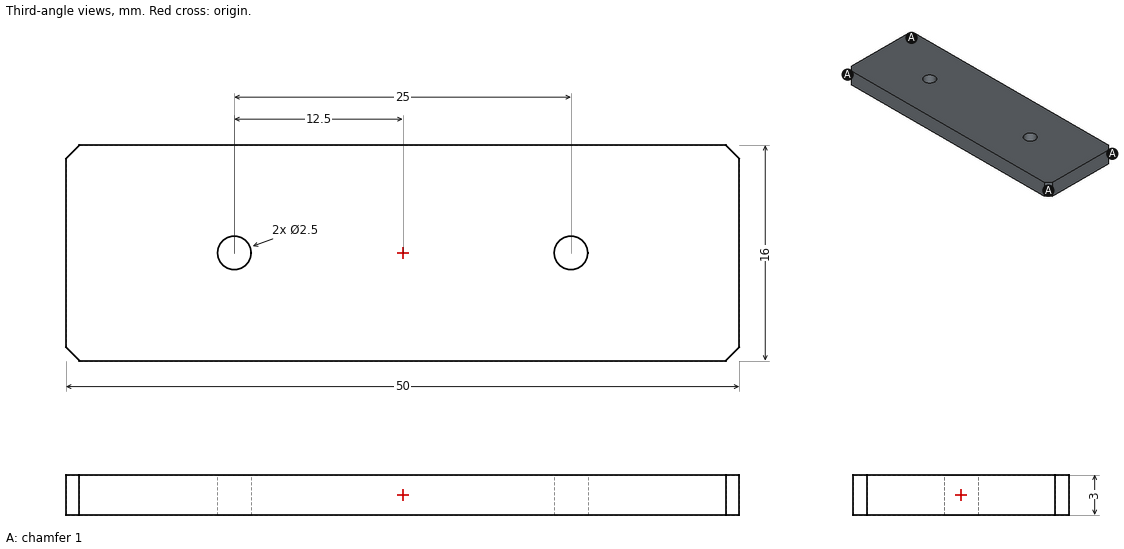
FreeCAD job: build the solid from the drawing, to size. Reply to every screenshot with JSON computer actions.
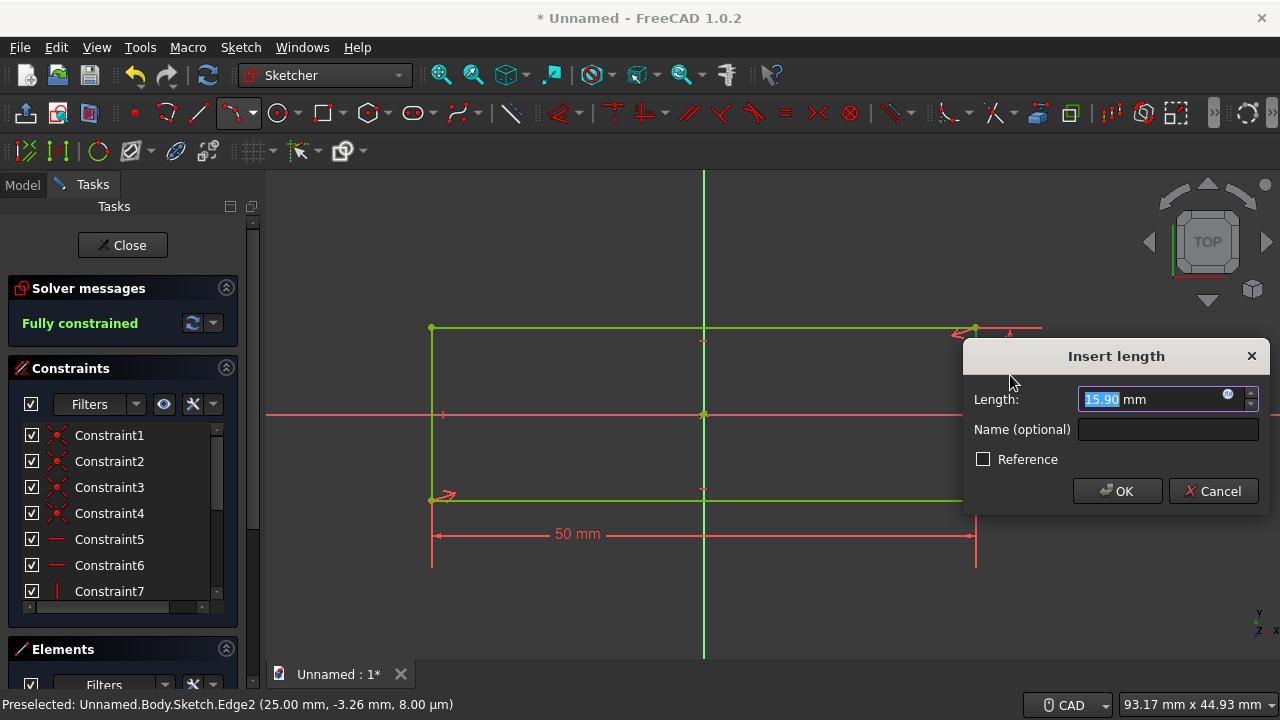
{"action": "type", "text": "16"}
{"action": "key", "text": "Return"}
{"action": "key", "text": "Escape"}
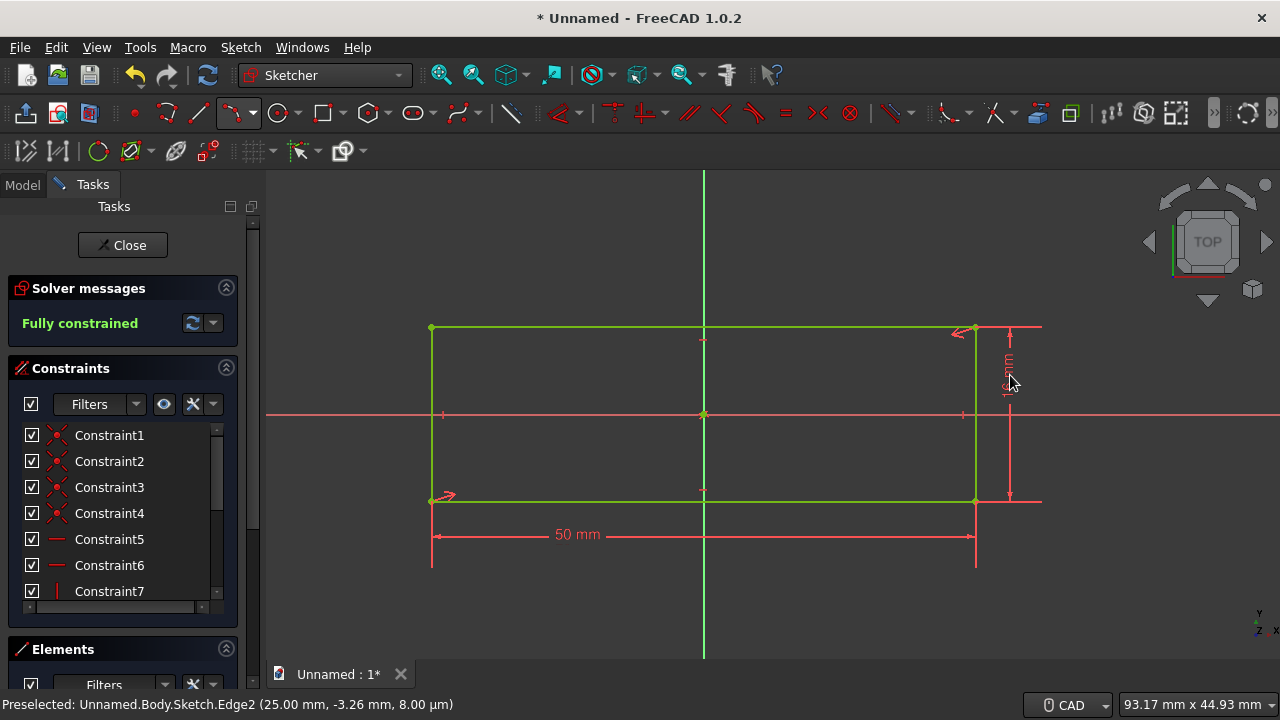
{"action": "left_click", "coordinate": [123, 245]}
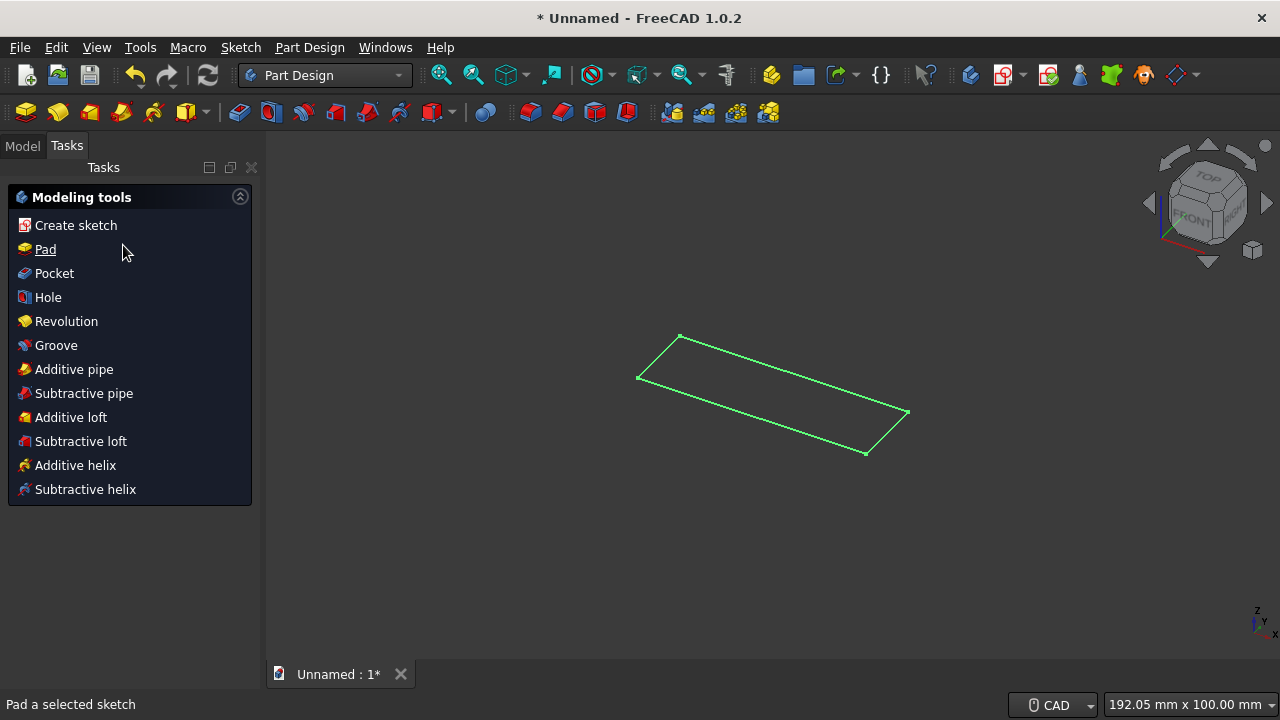
{"action": "left_click", "coordinate": [26, 112]}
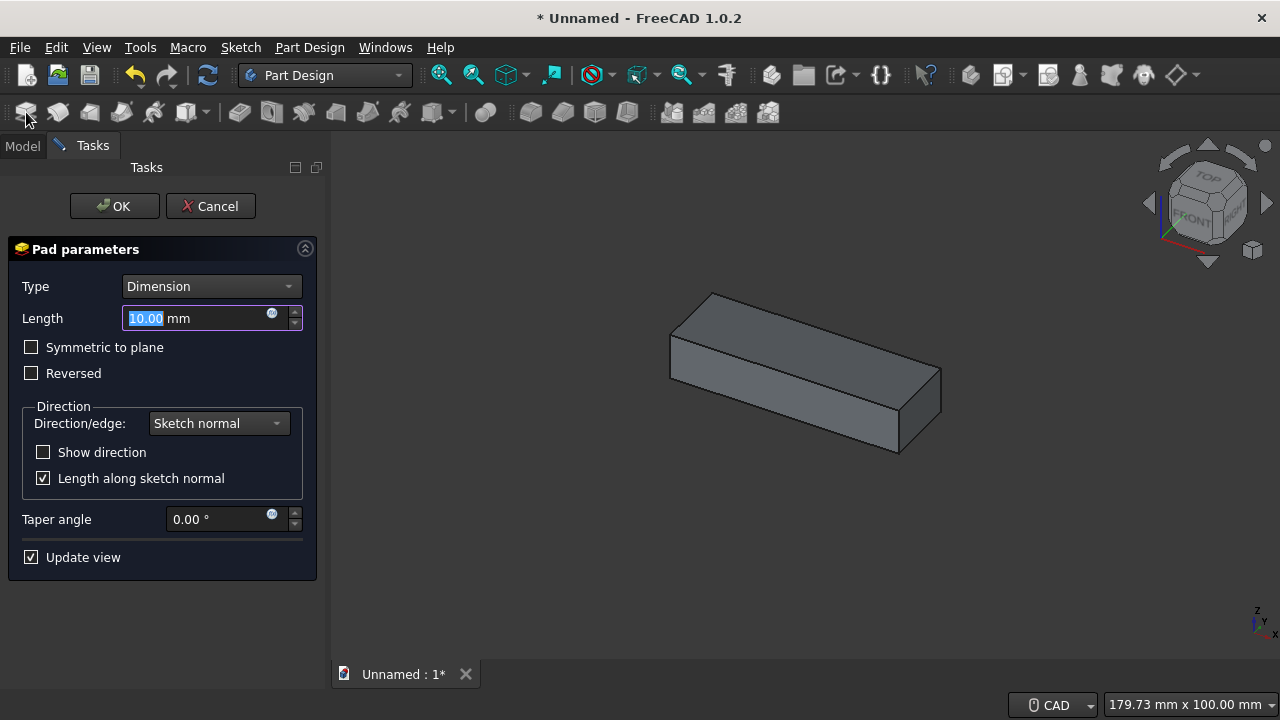
{"action": "type", "text": "3"}
{"action": "key", "text": "Tab"}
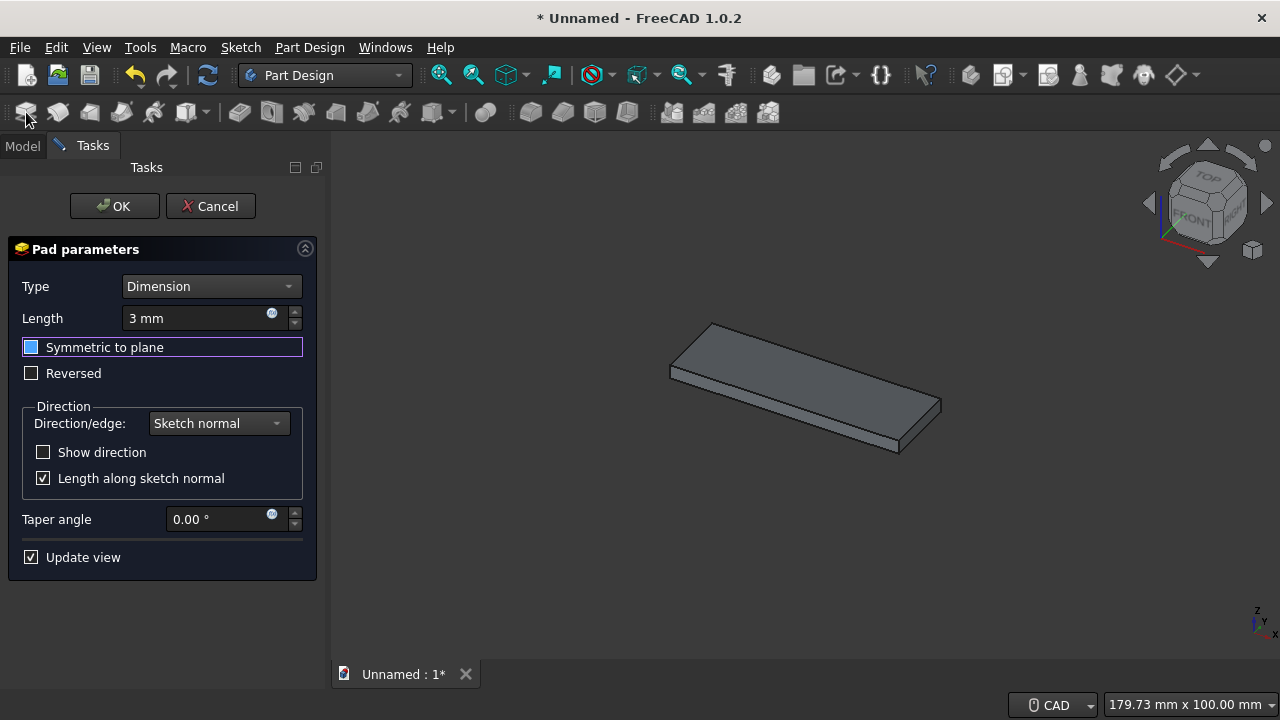
{"action": "left_click", "coordinate": [30, 347]}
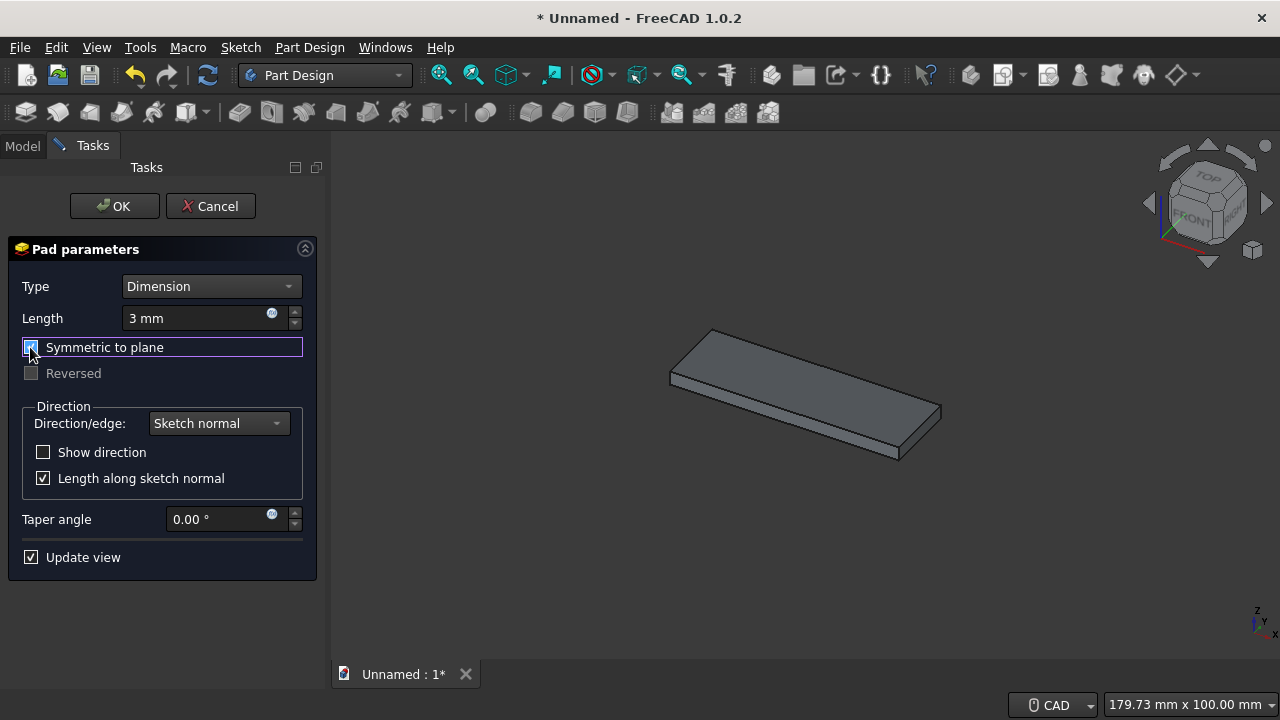
{"action": "left_click", "coordinate": [115, 206]}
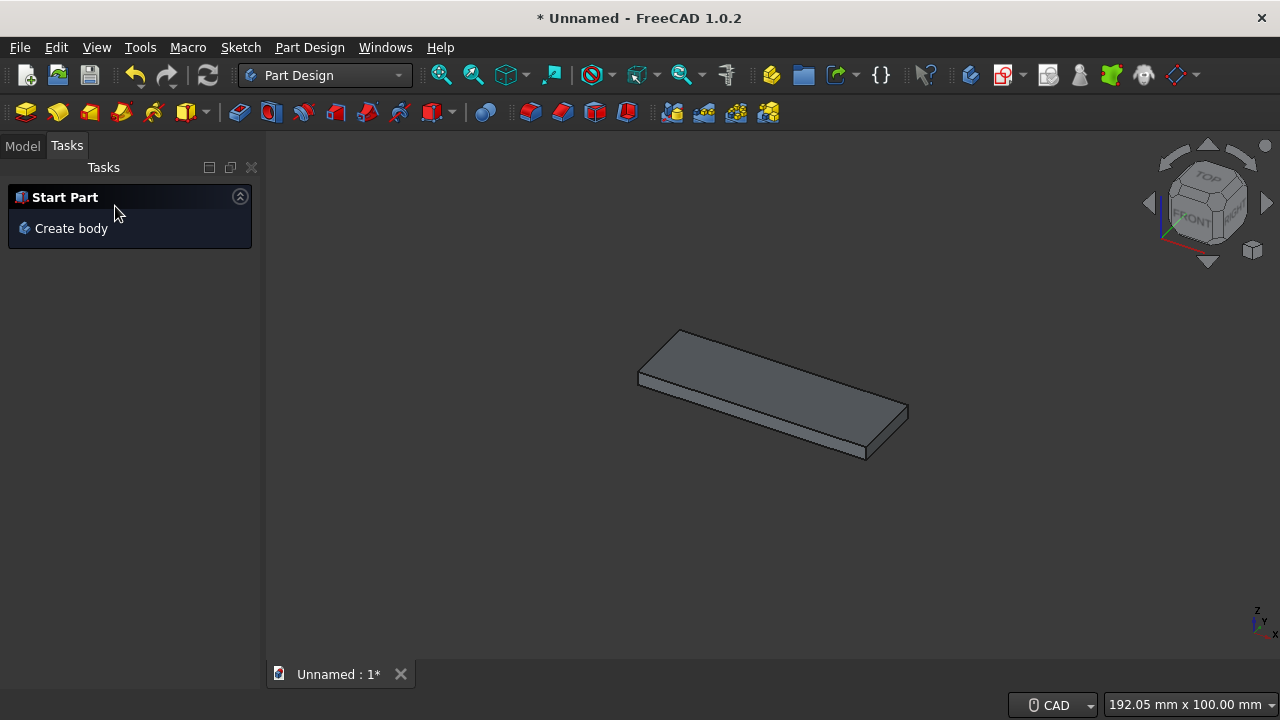
{"action": "left_click", "coordinate": [442, 76]}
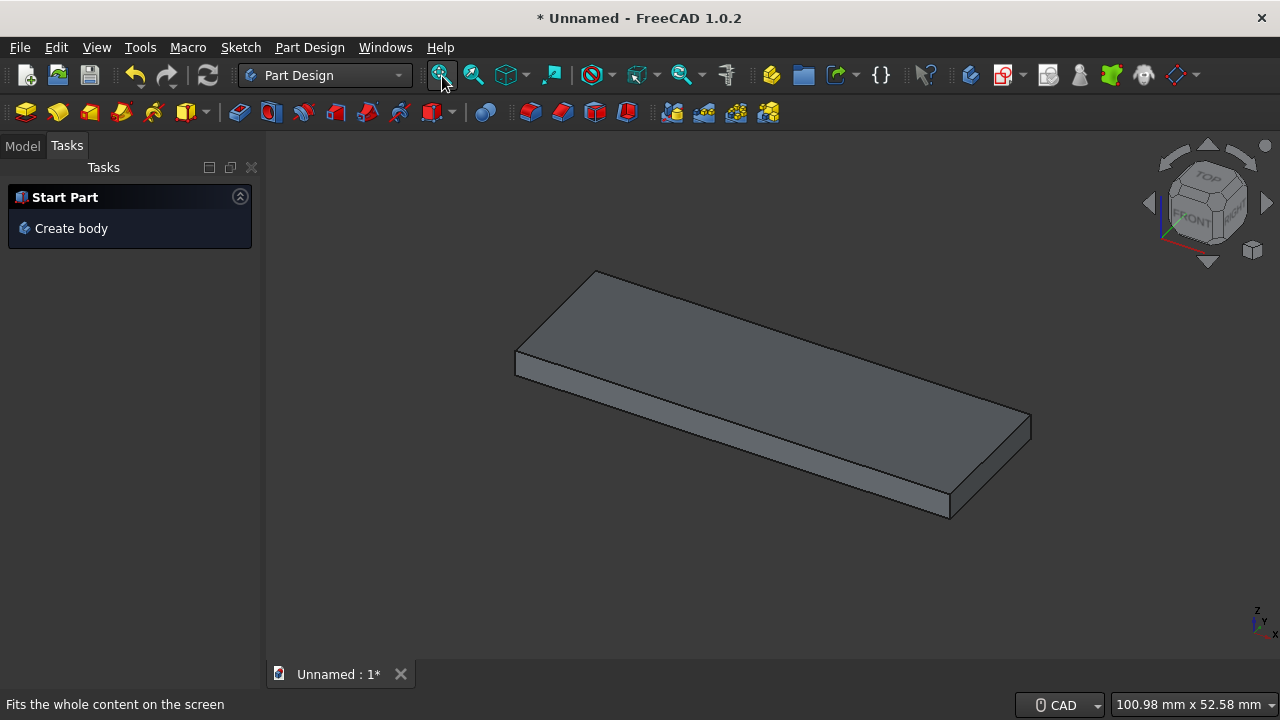
{"action": "key", "text": "5"}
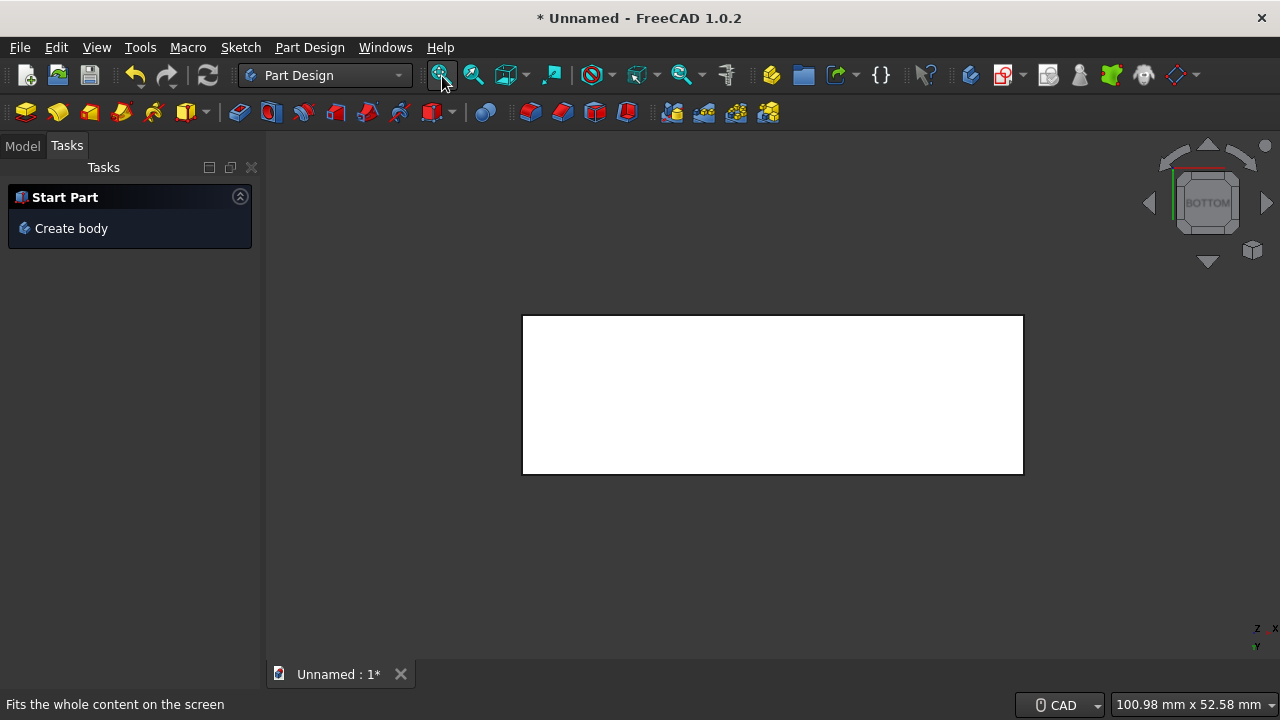
{"action": "left_click", "coordinate": [916, 394]}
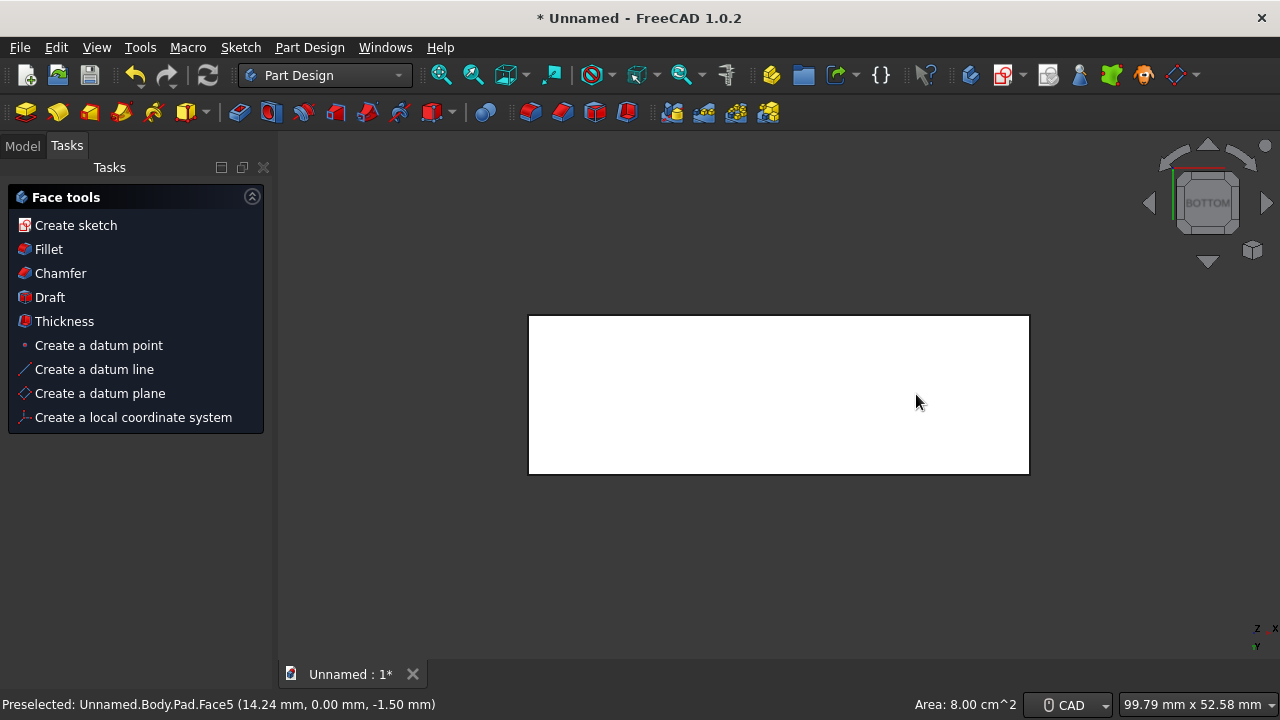
{"action": "left_click", "coordinate": [1004, 76]}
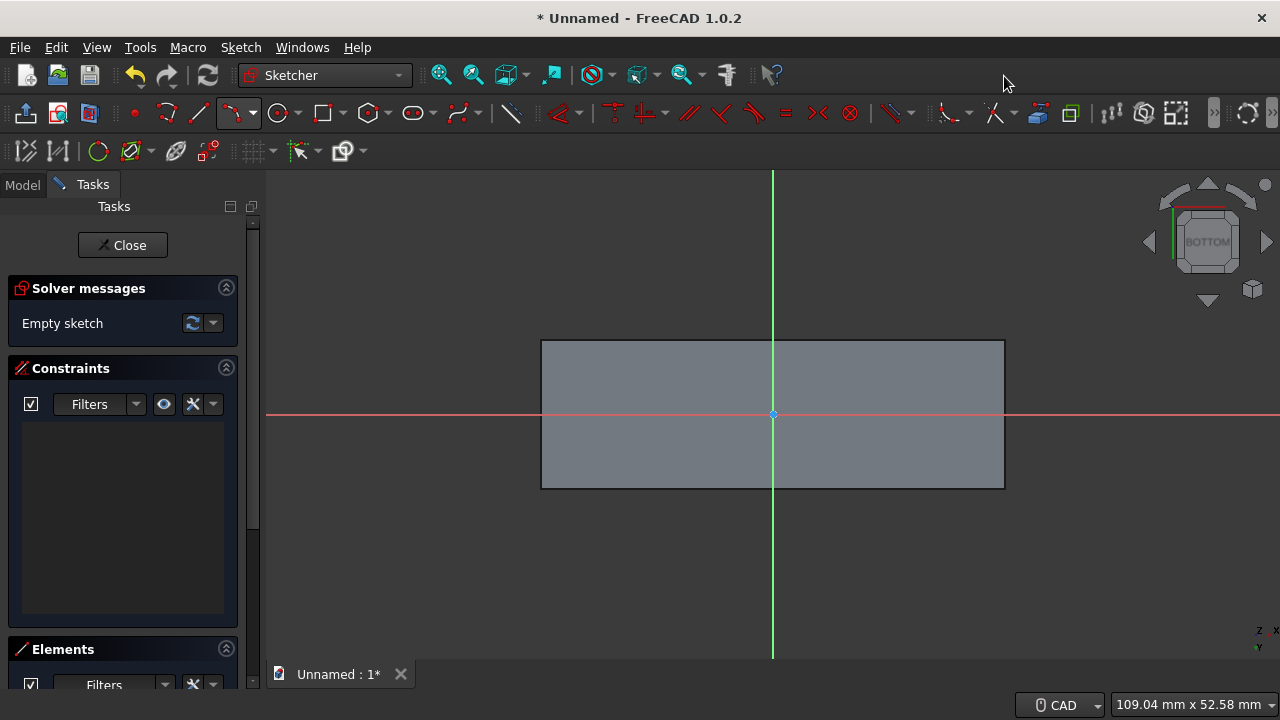
{"action": "scroll", "coordinate": [829, 414], "scroll_direction": "up", "scroll_amount": 4}